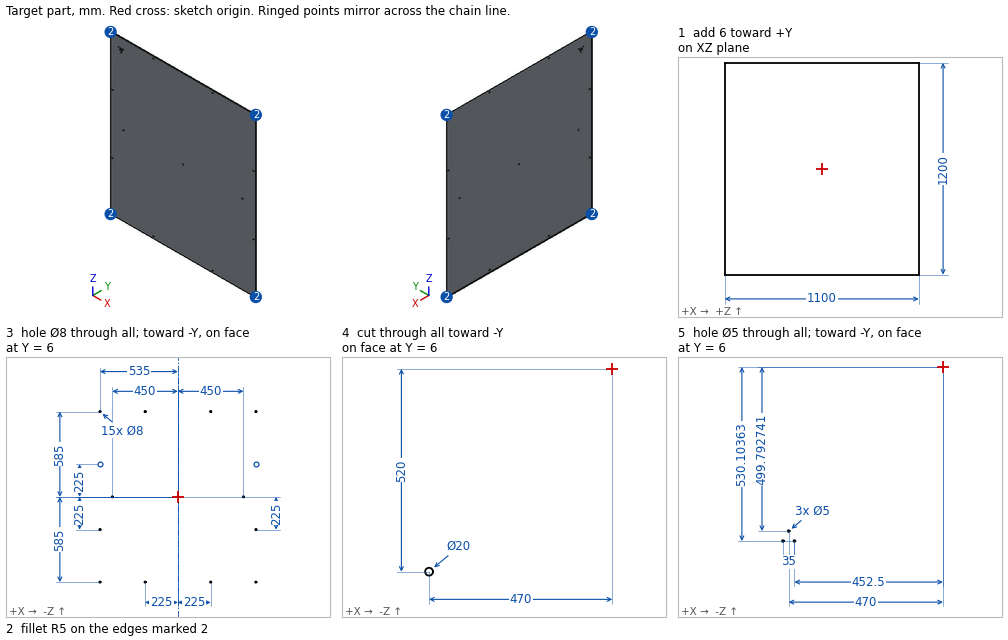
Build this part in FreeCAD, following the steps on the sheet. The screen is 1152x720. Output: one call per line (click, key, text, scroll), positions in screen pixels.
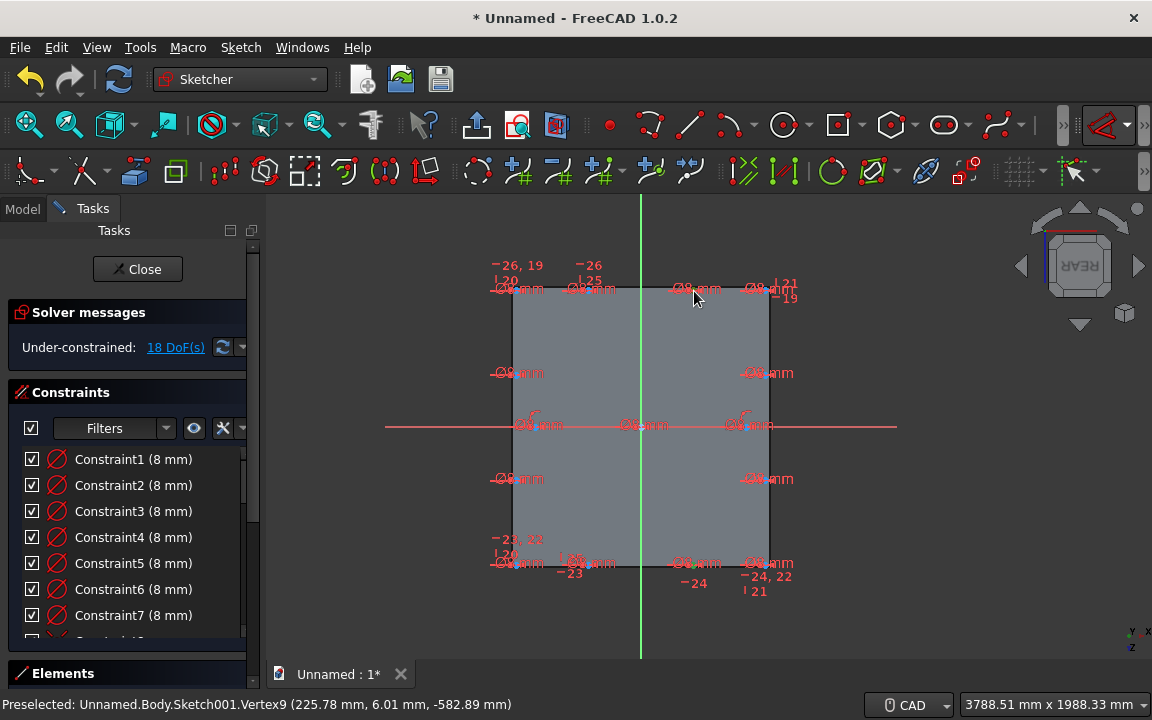
key(v)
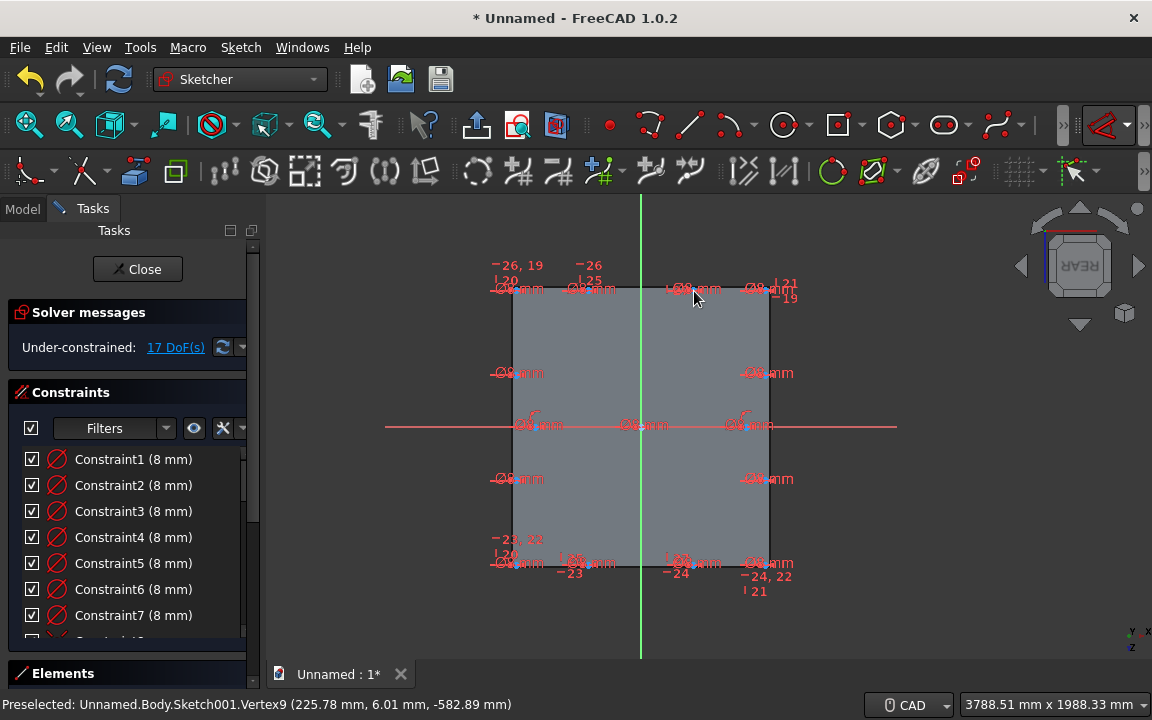
click(766, 291)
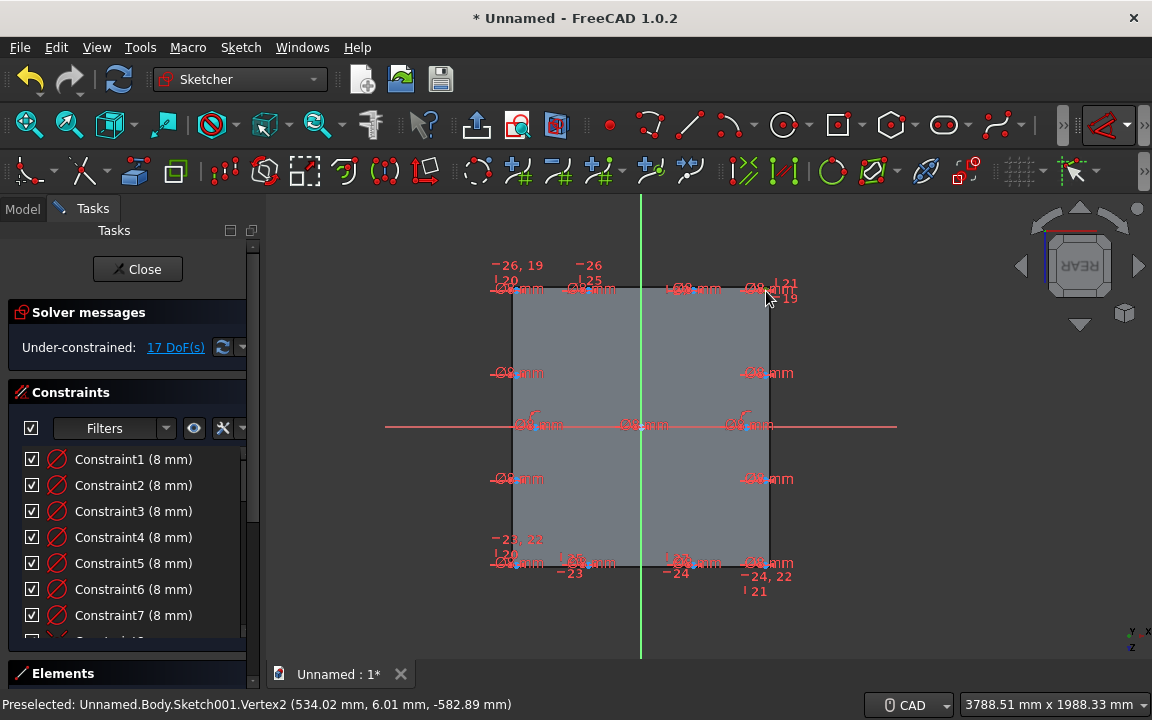
click(694, 291)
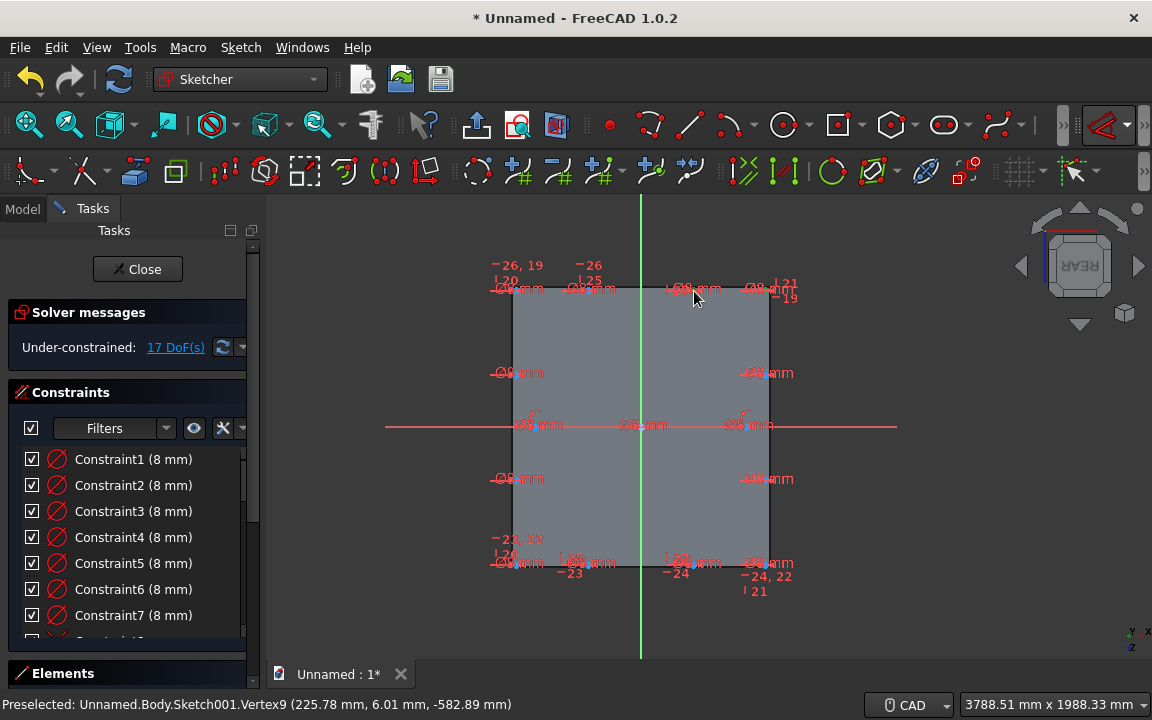
key(h)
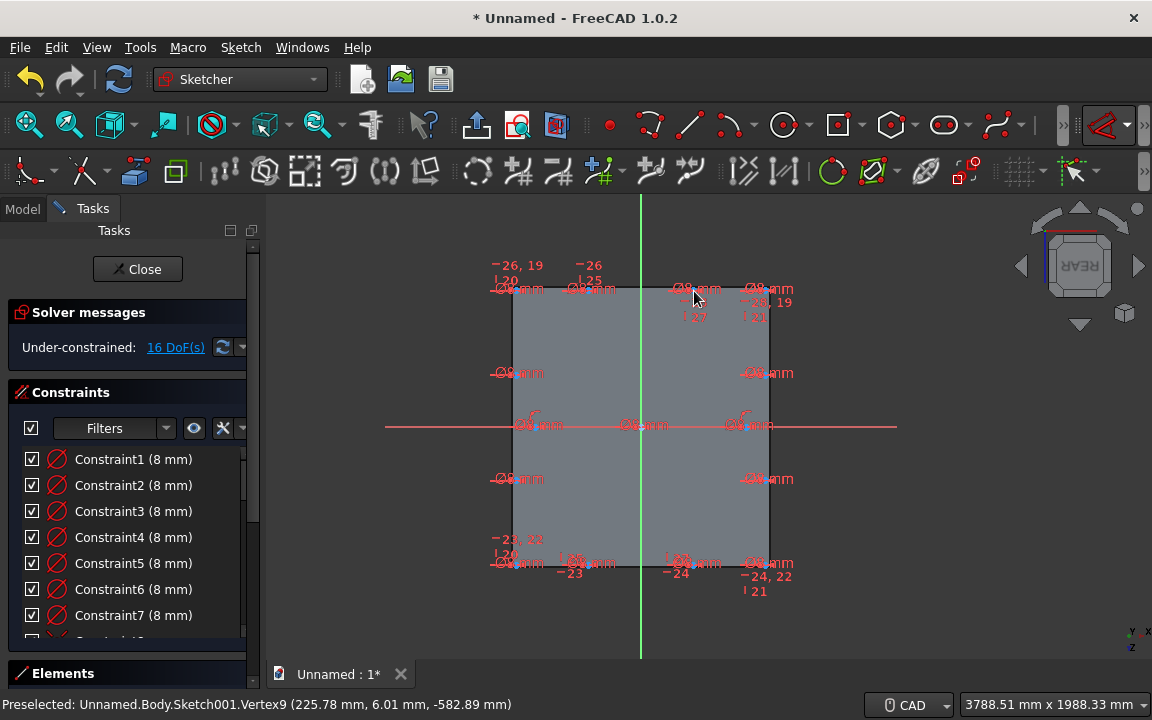
click(516, 565)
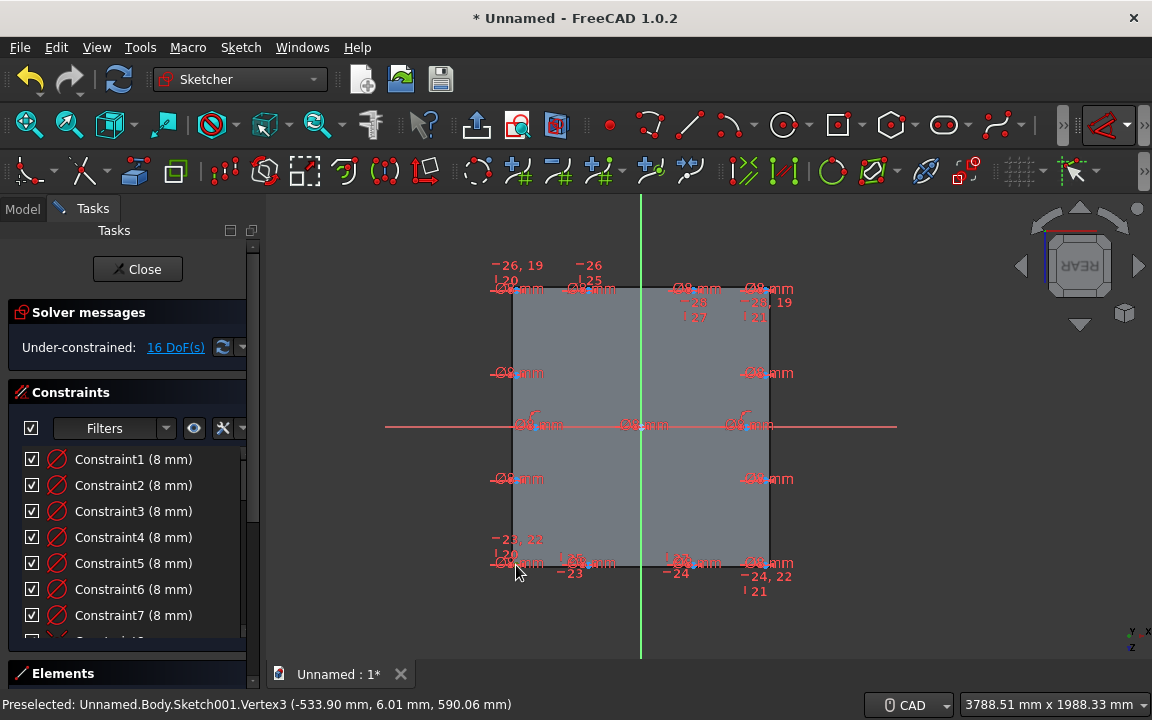
click(516, 481)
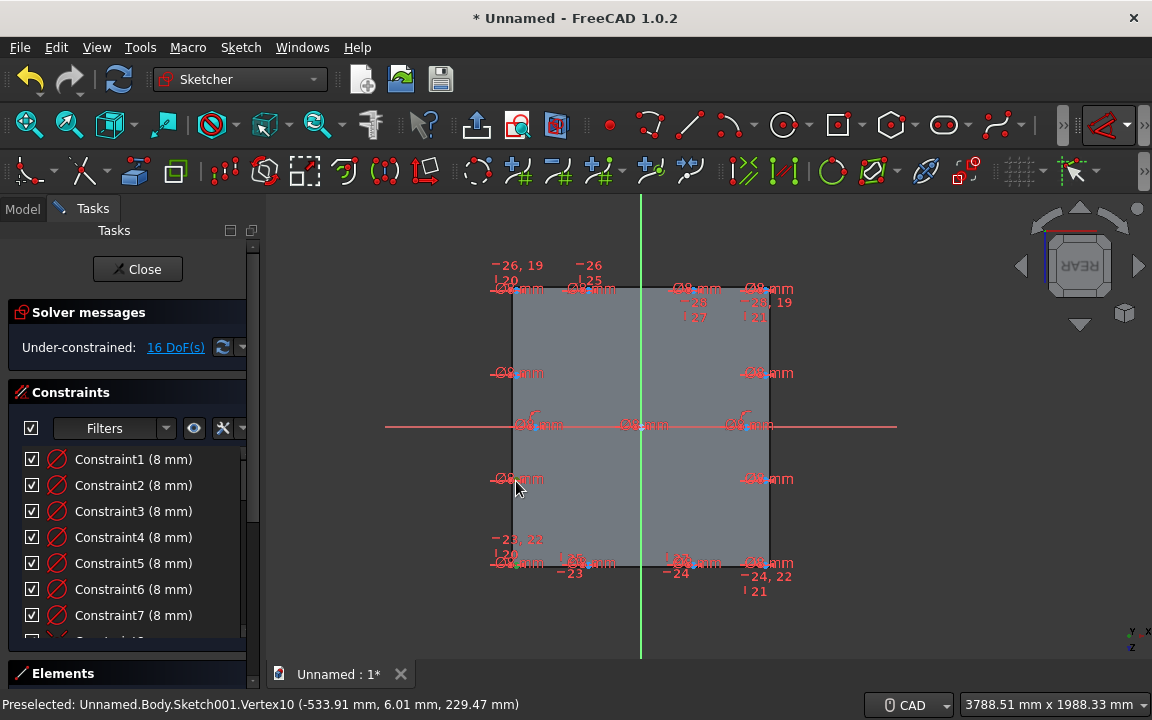
key(v)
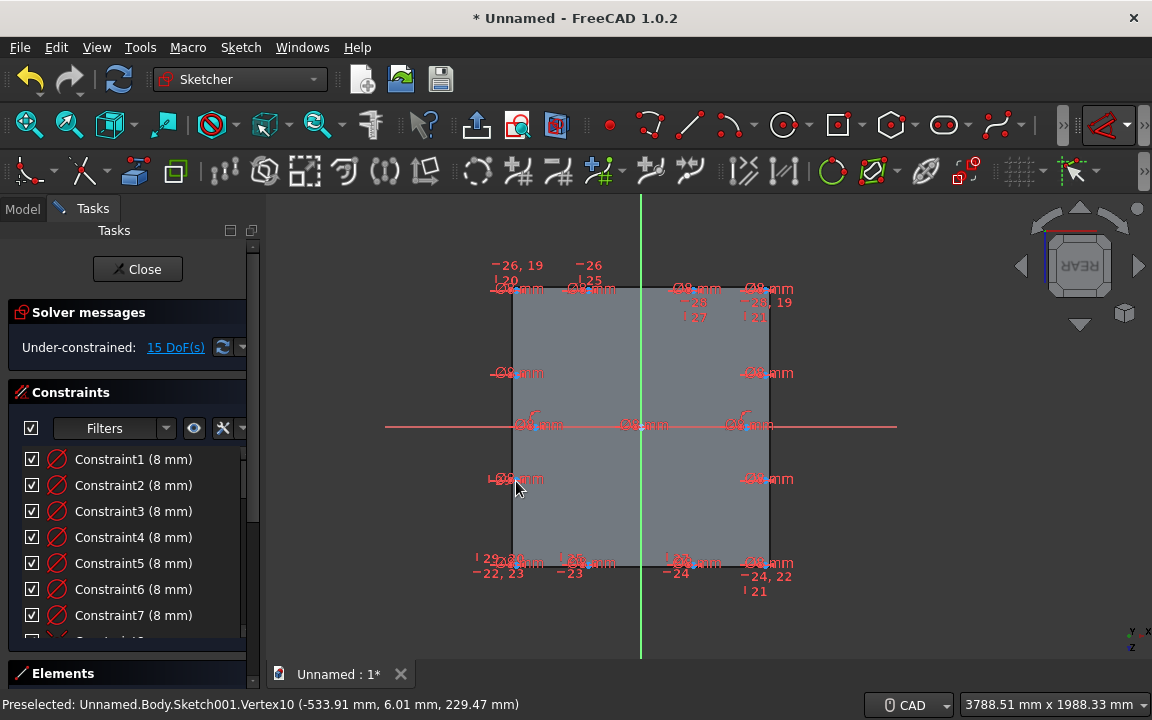
click(516, 291)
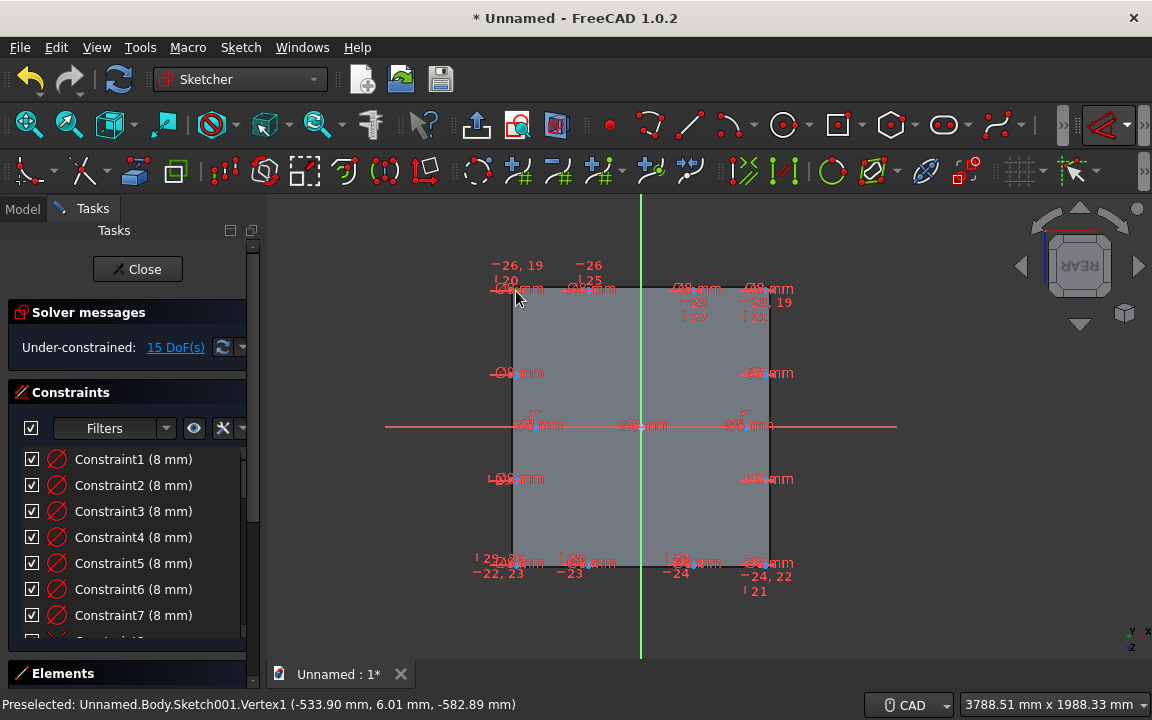
click(516, 375)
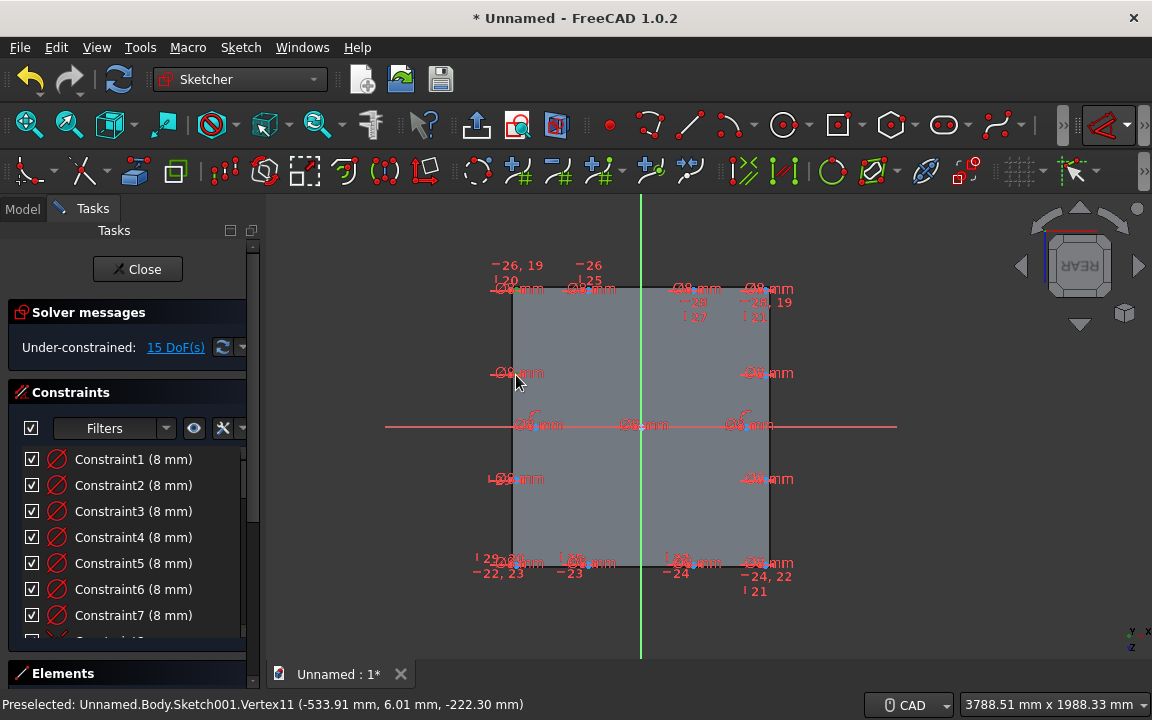
key(v)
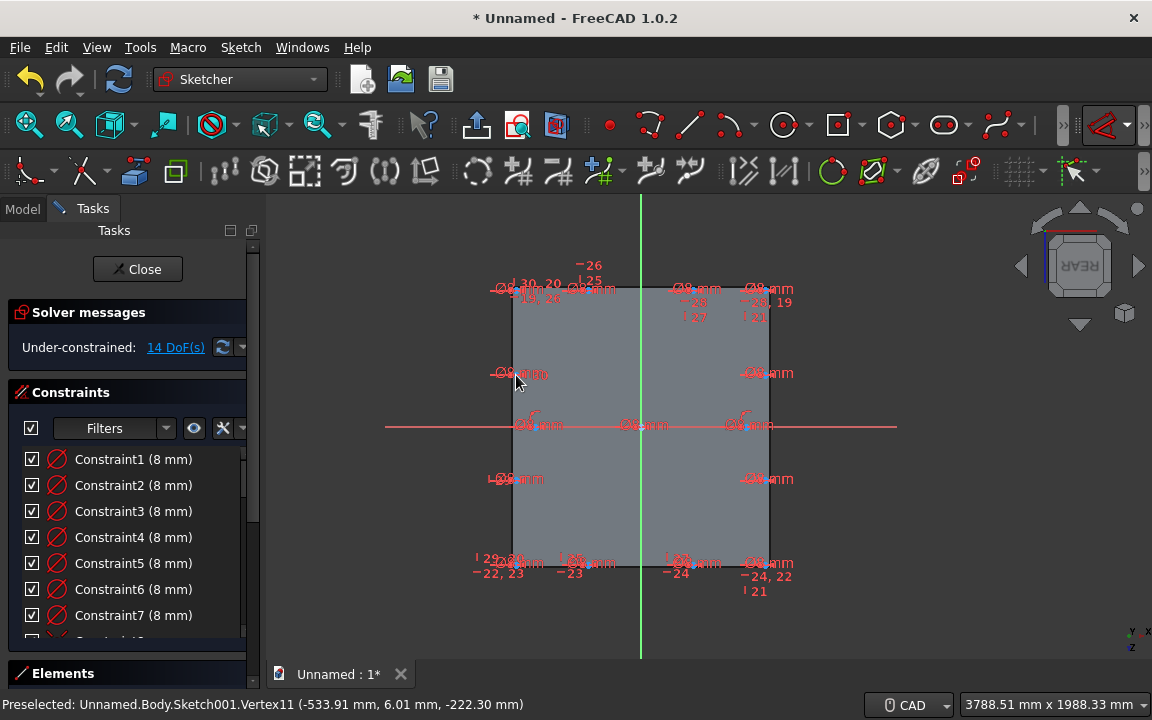
click(766, 291)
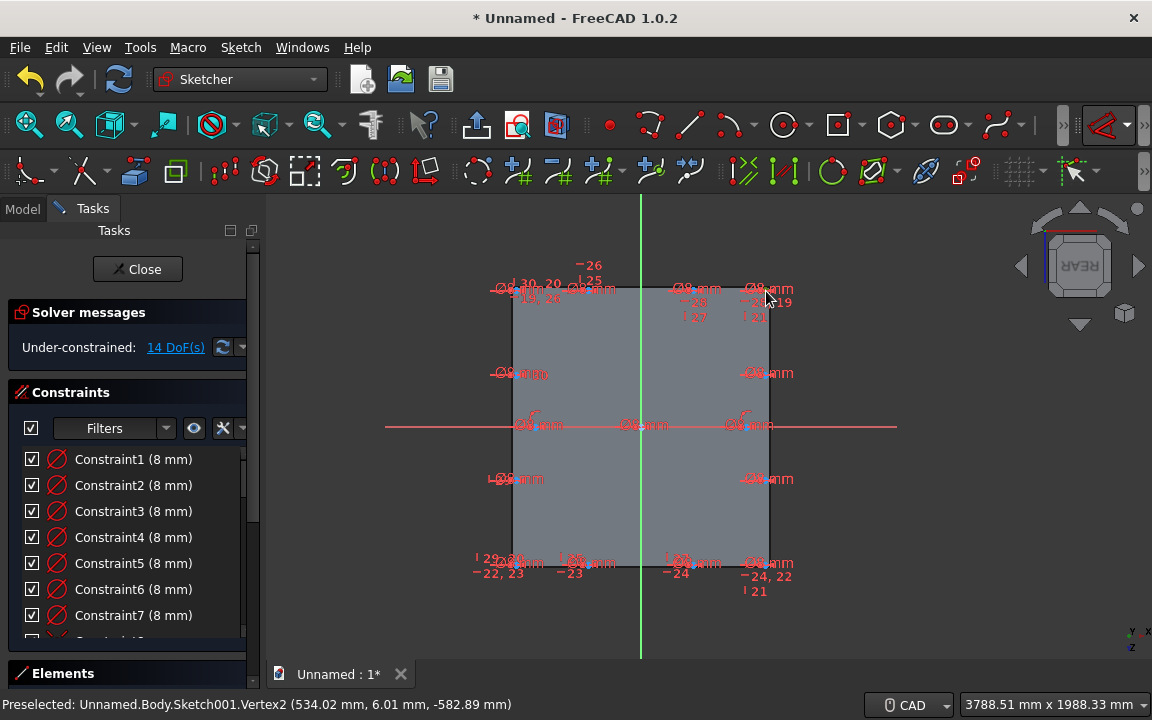
click(766, 375)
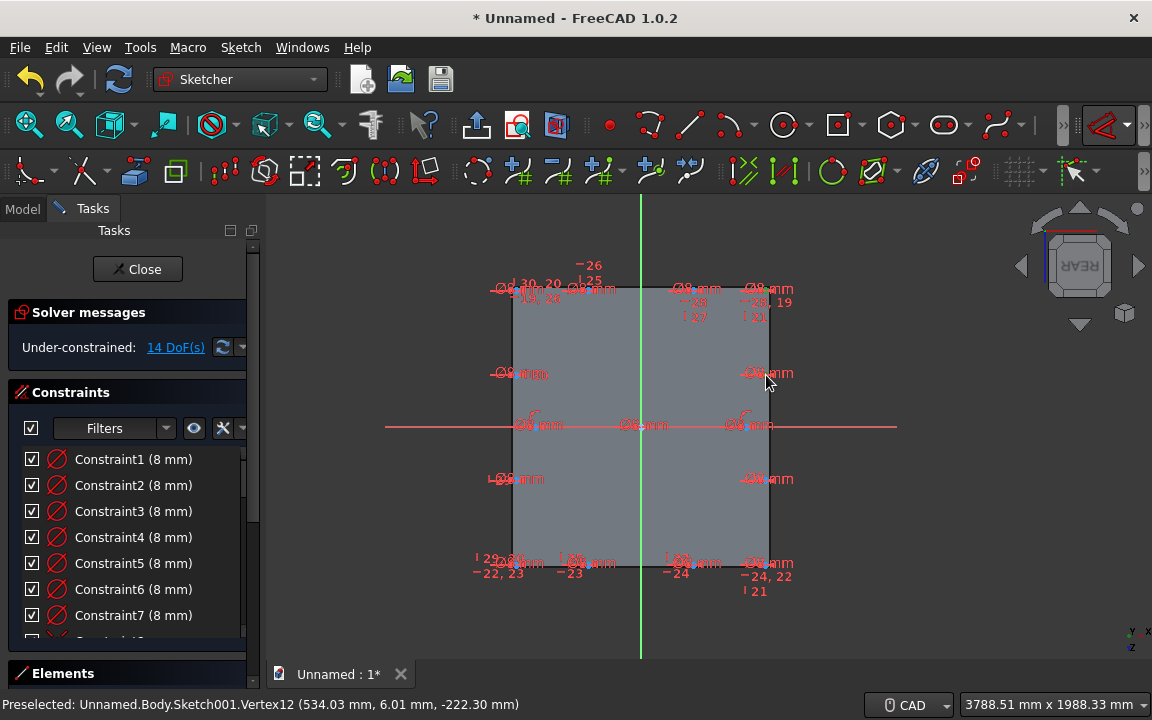
key(v)